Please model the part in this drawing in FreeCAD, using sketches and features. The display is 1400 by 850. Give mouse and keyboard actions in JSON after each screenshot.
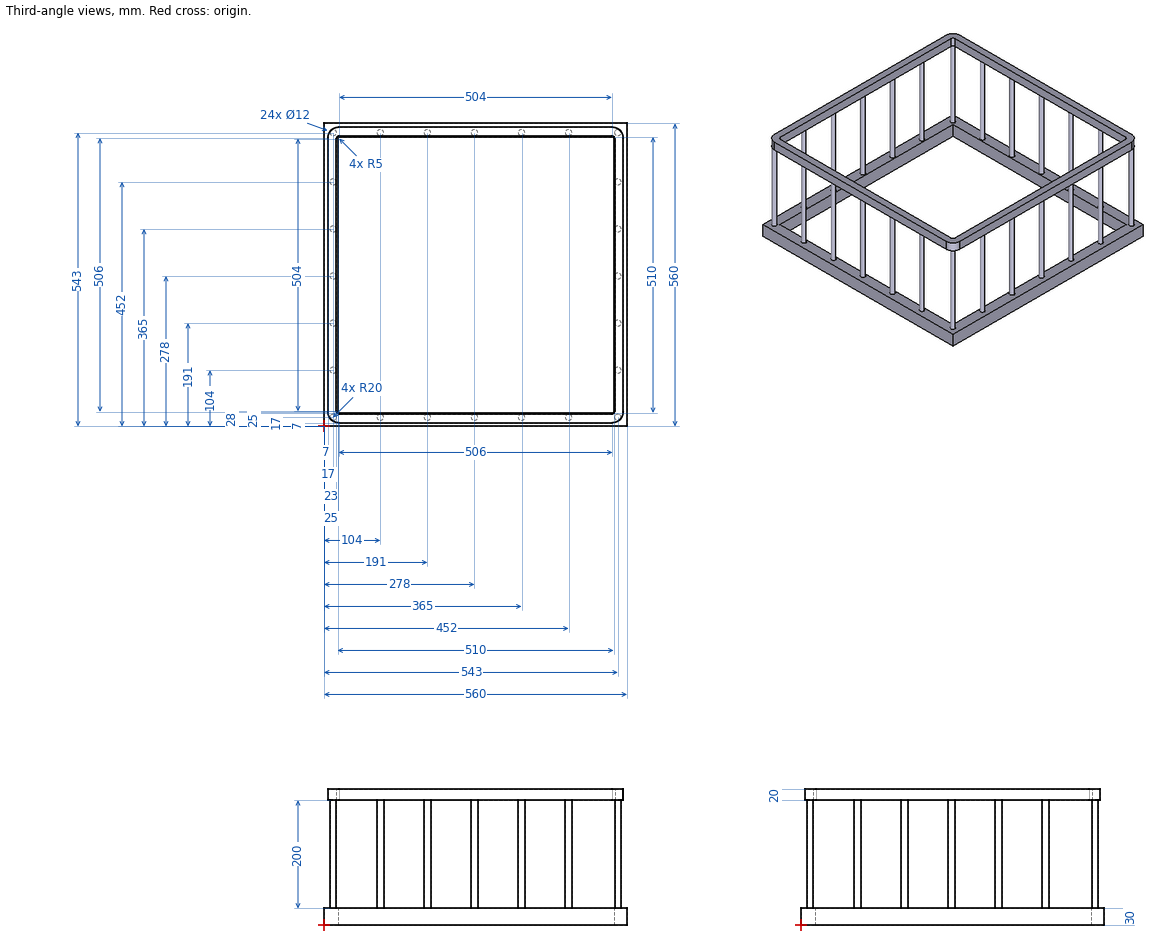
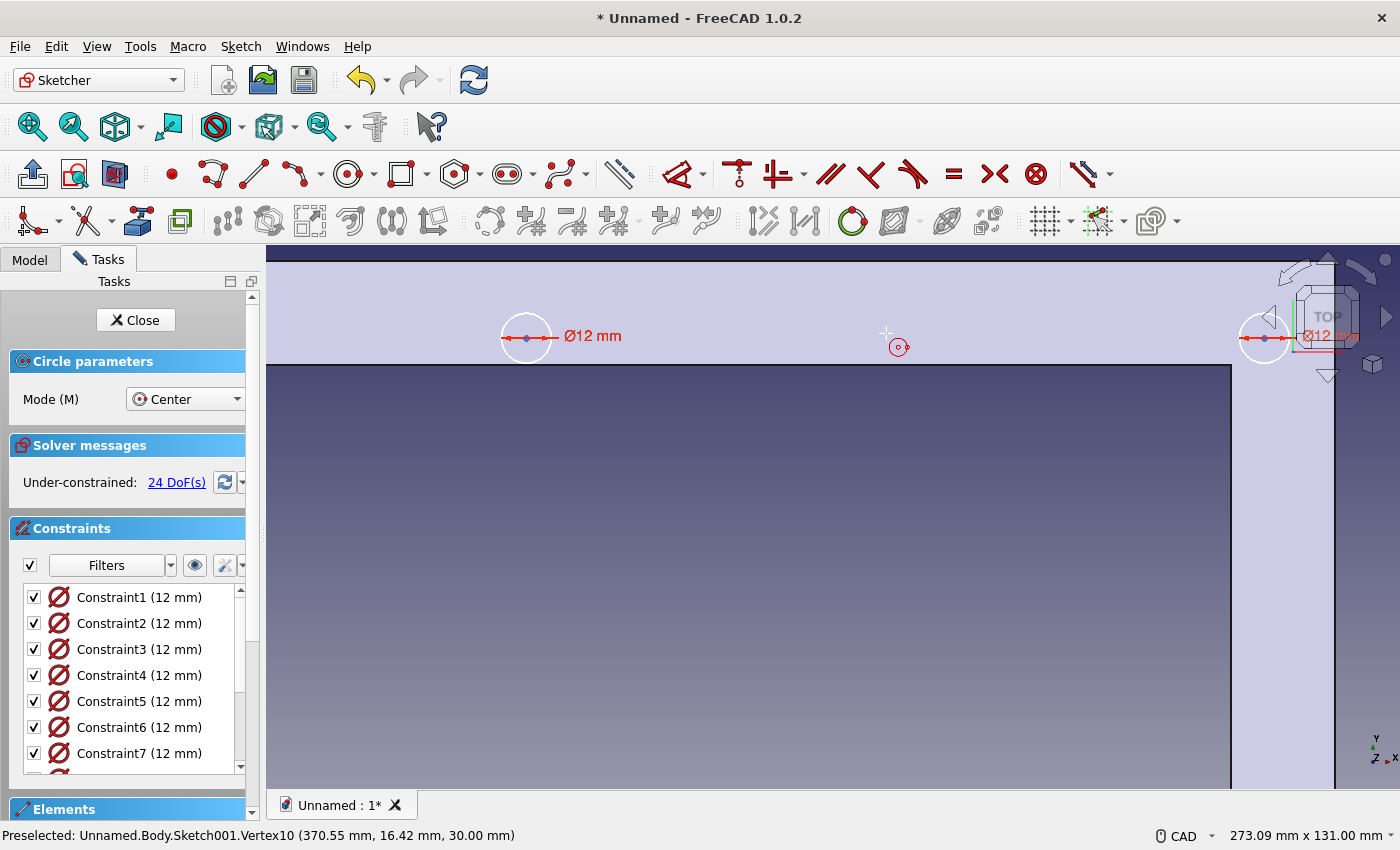
{"action": "scroll", "coordinate": [886, 333], "scroll_direction": "down", "scroll_amount": 9}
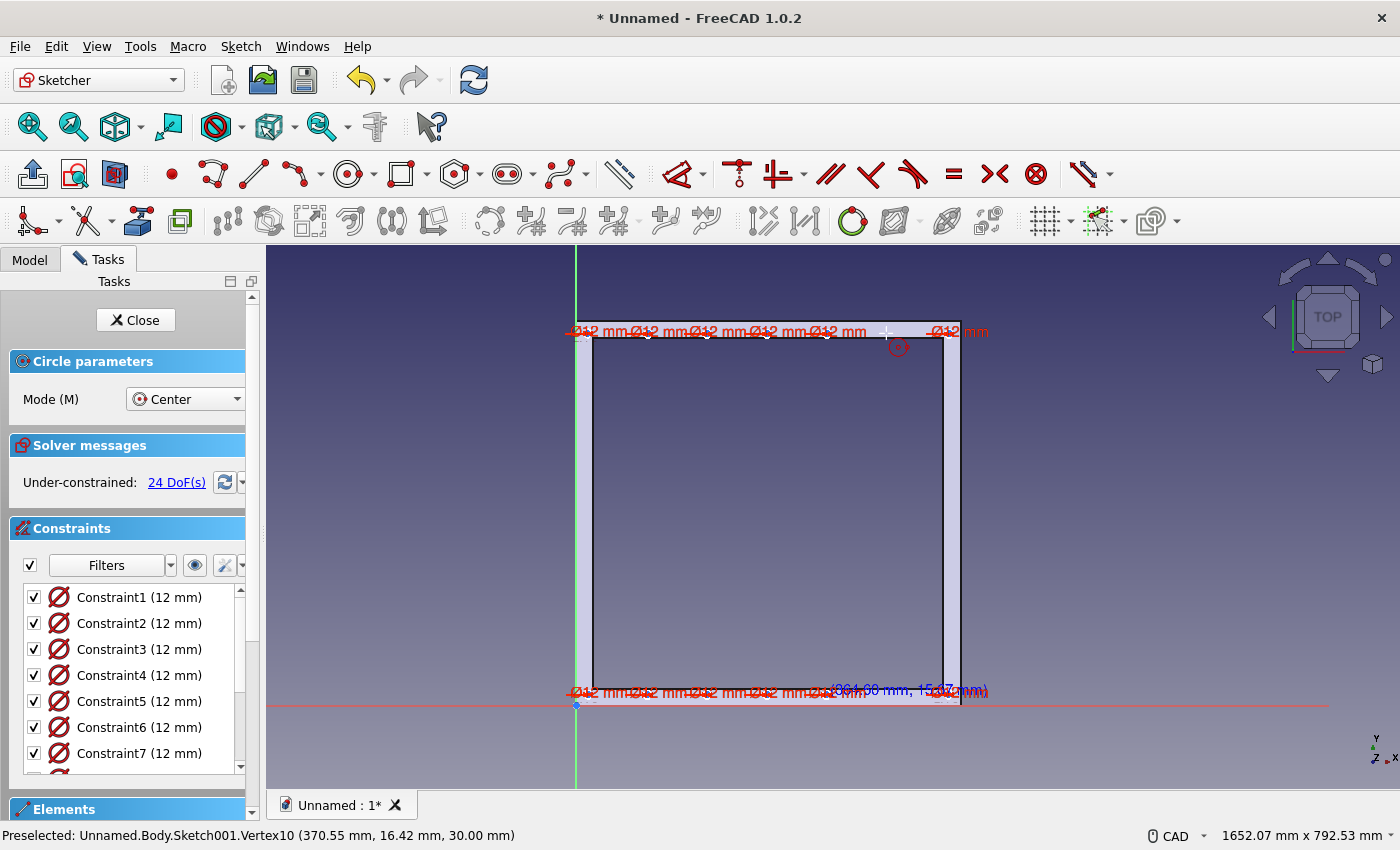
{"action": "left_click", "coordinate": [886, 333]}
{"action": "mouse_move", "coordinate": [889, 330]}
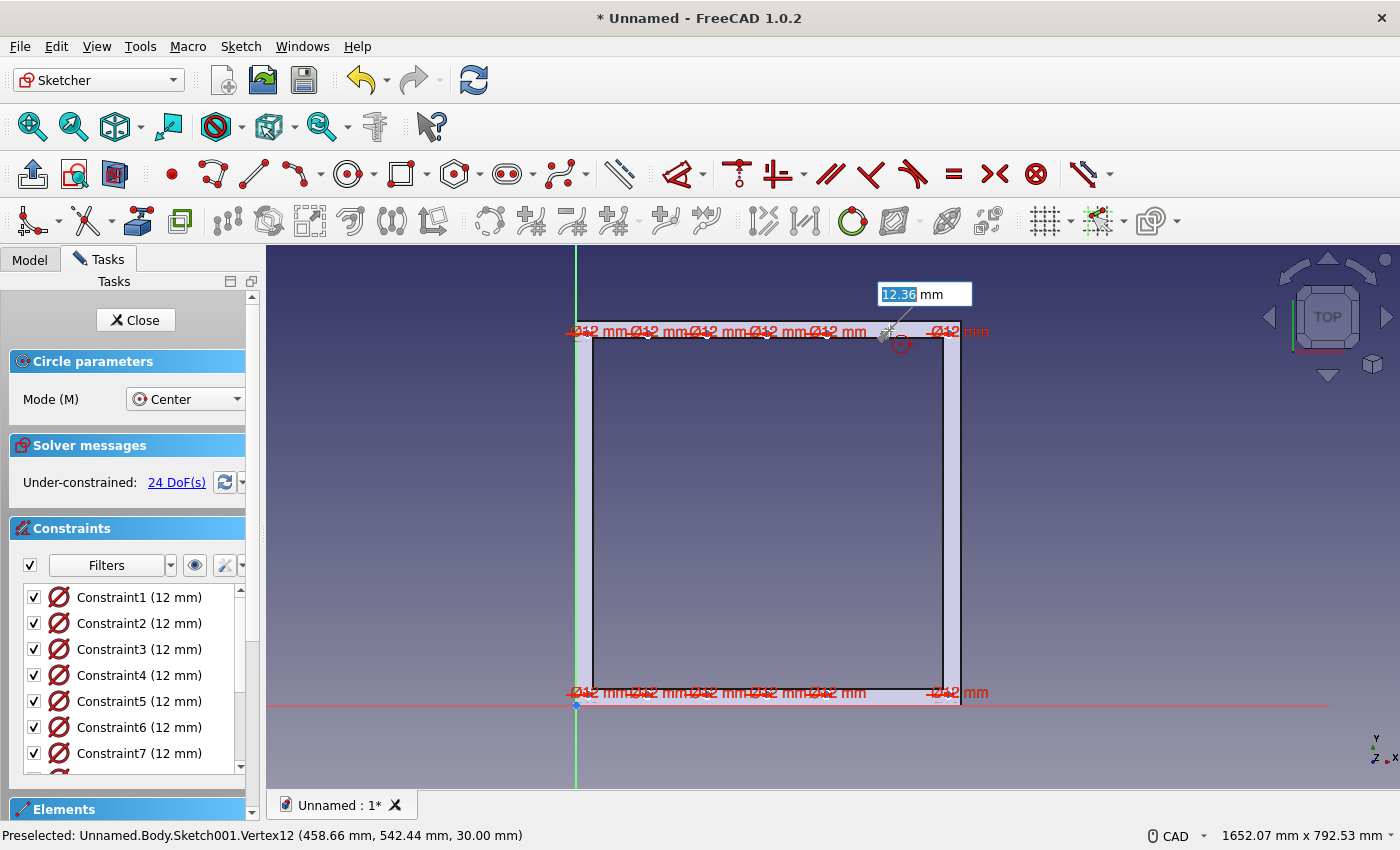
{"action": "type", "text": "12"}
{"action": "key", "text": "Return"}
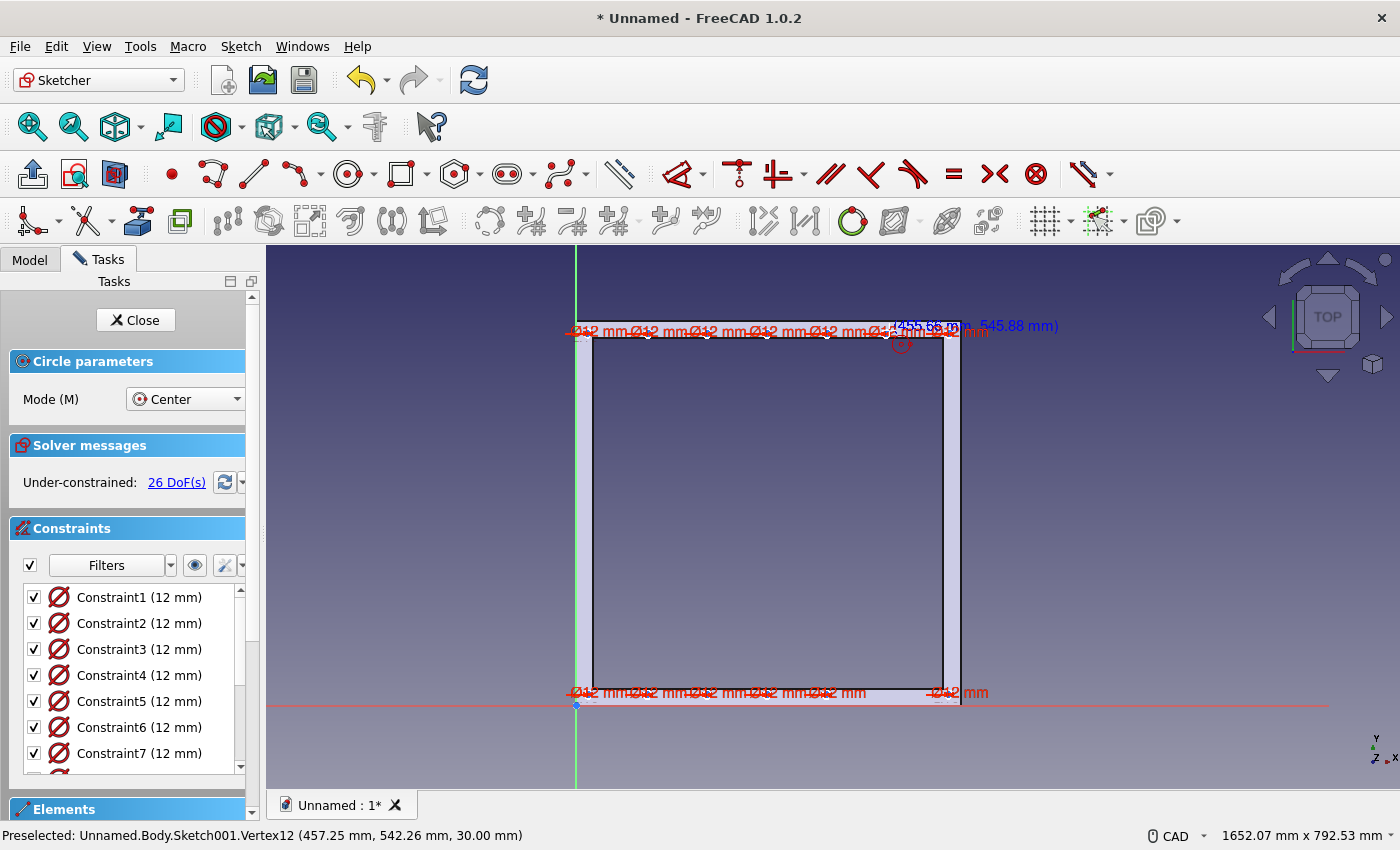
{"action": "scroll", "coordinate": [886, 694], "scroll_direction": "up", "scroll_amount": 9}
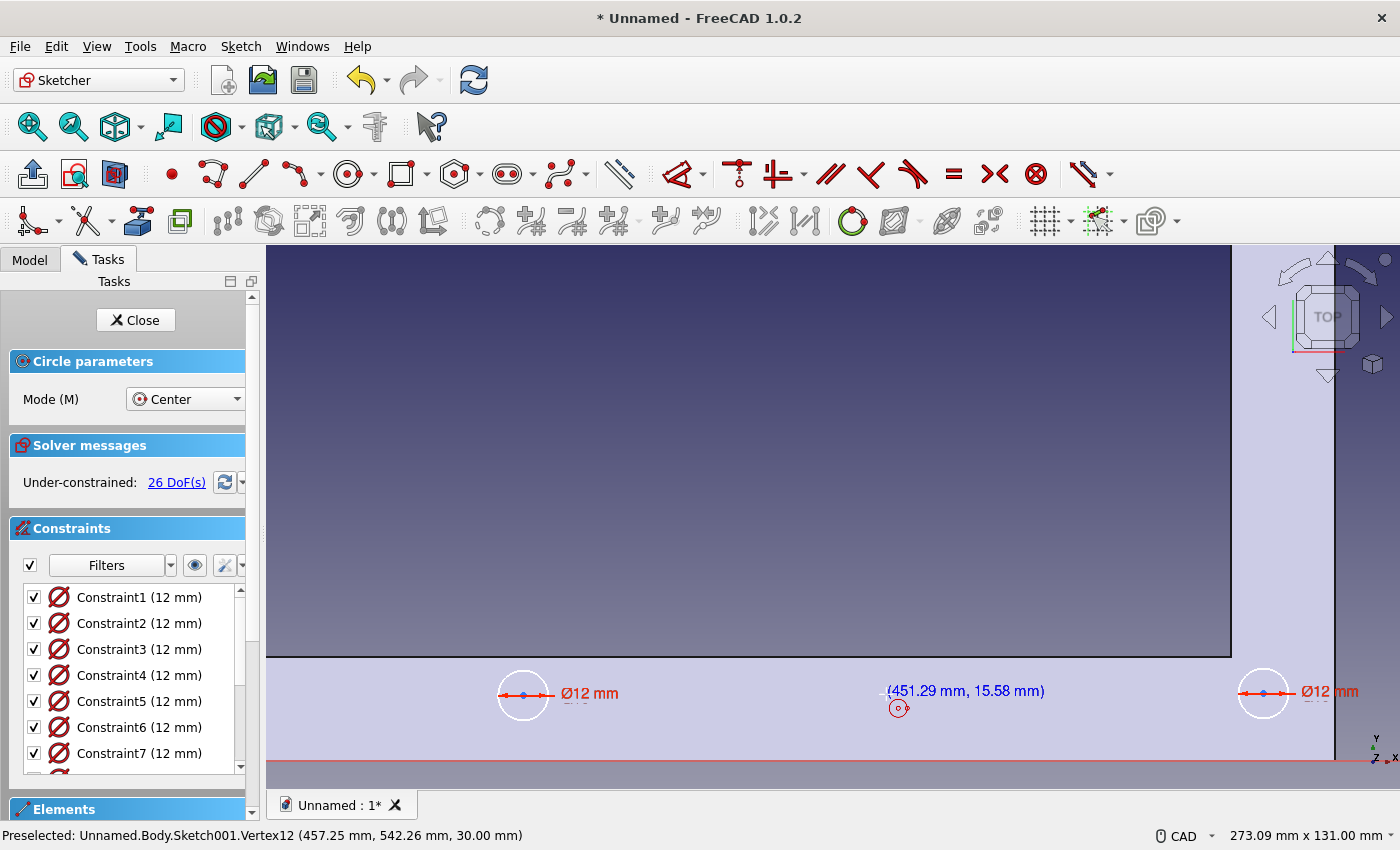
{"action": "scroll", "coordinate": [886, 694], "scroll_direction": "down", "scroll_amount": 9}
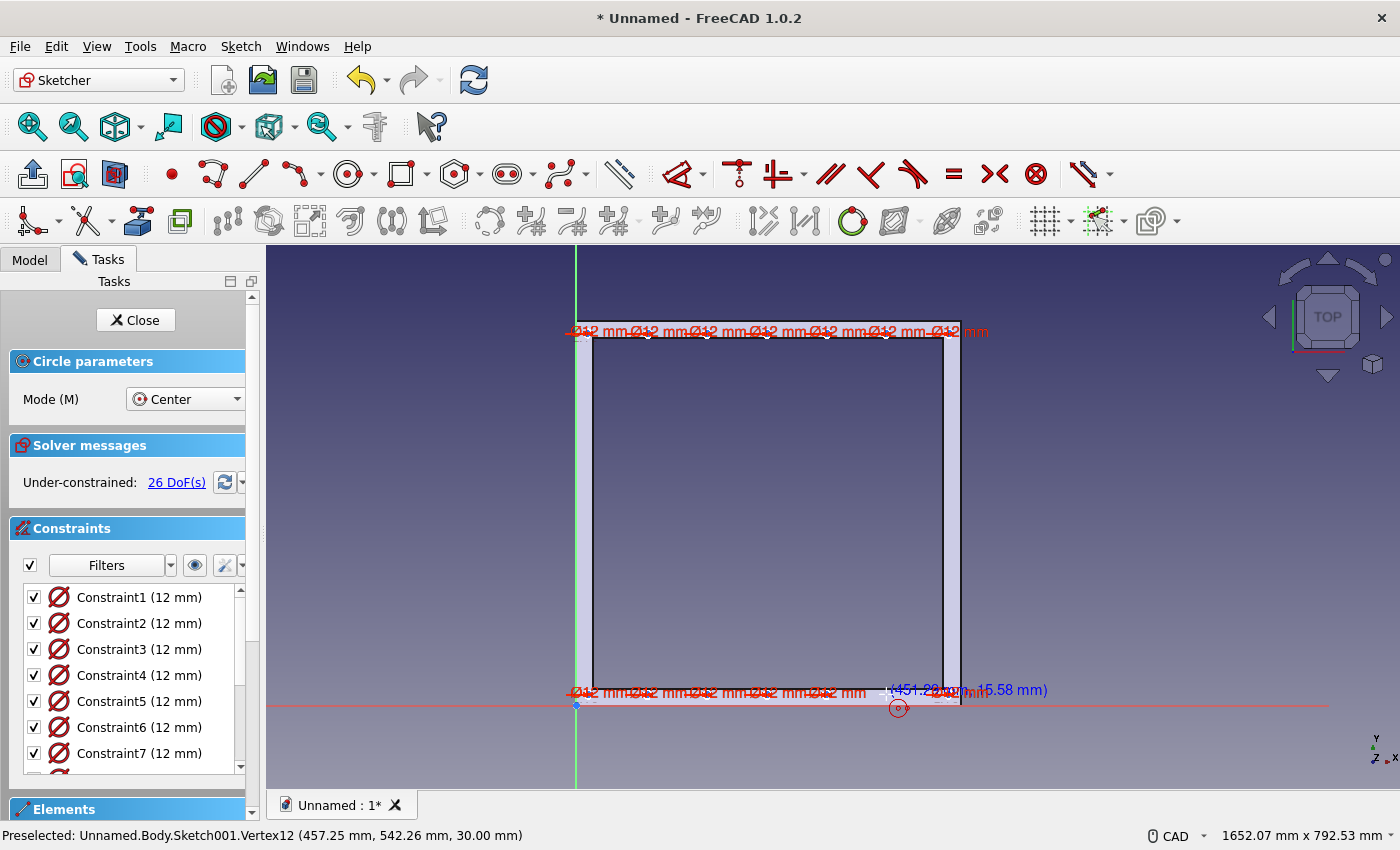
{"action": "scroll", "coordinate": [886, 694], "scroll_direction": "up", "scroll_amount": 2}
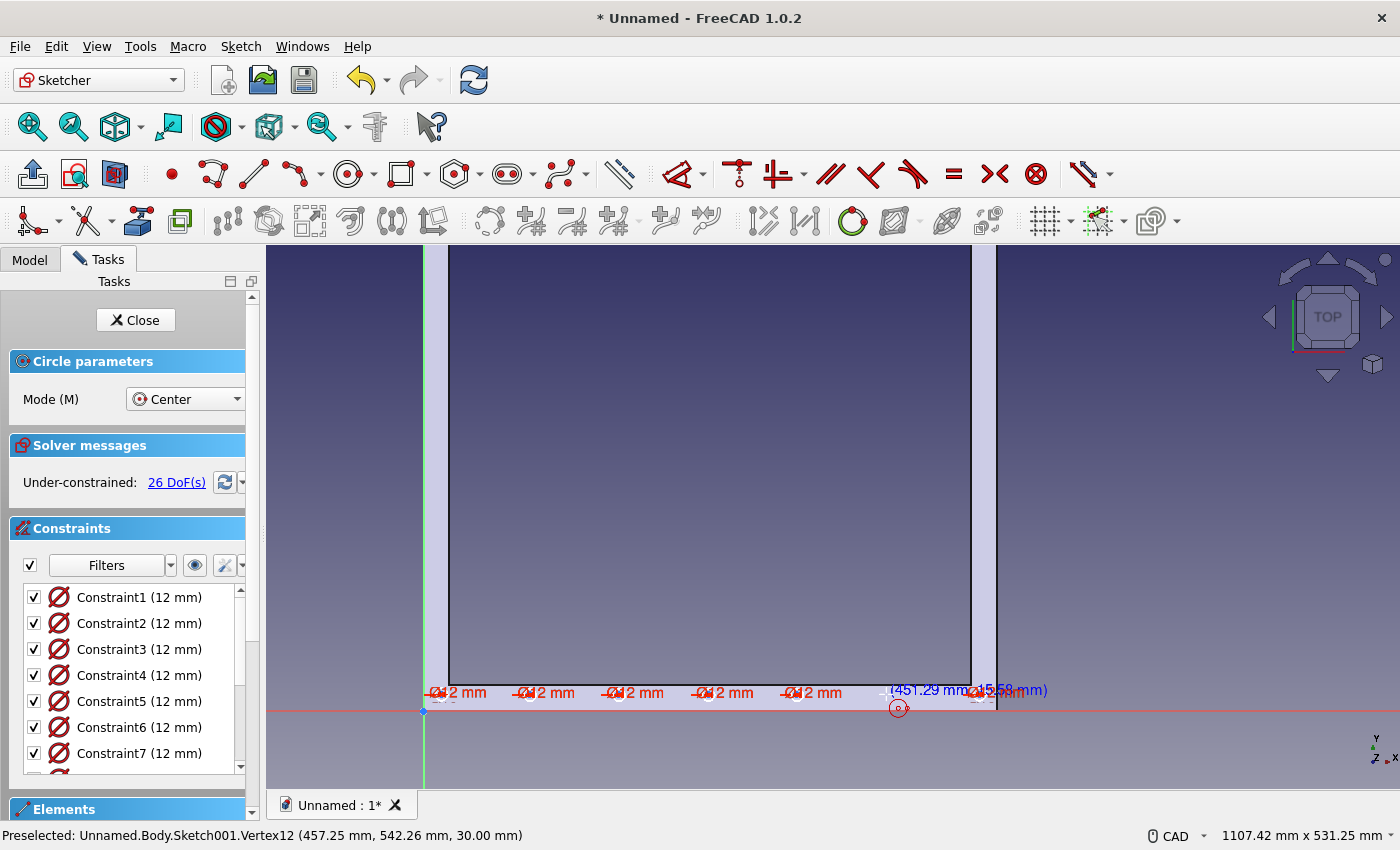
{"action": "left_click", "coordinate": [886, 694]}
{"action": "mouse_move", "coordinate": [891, 689]}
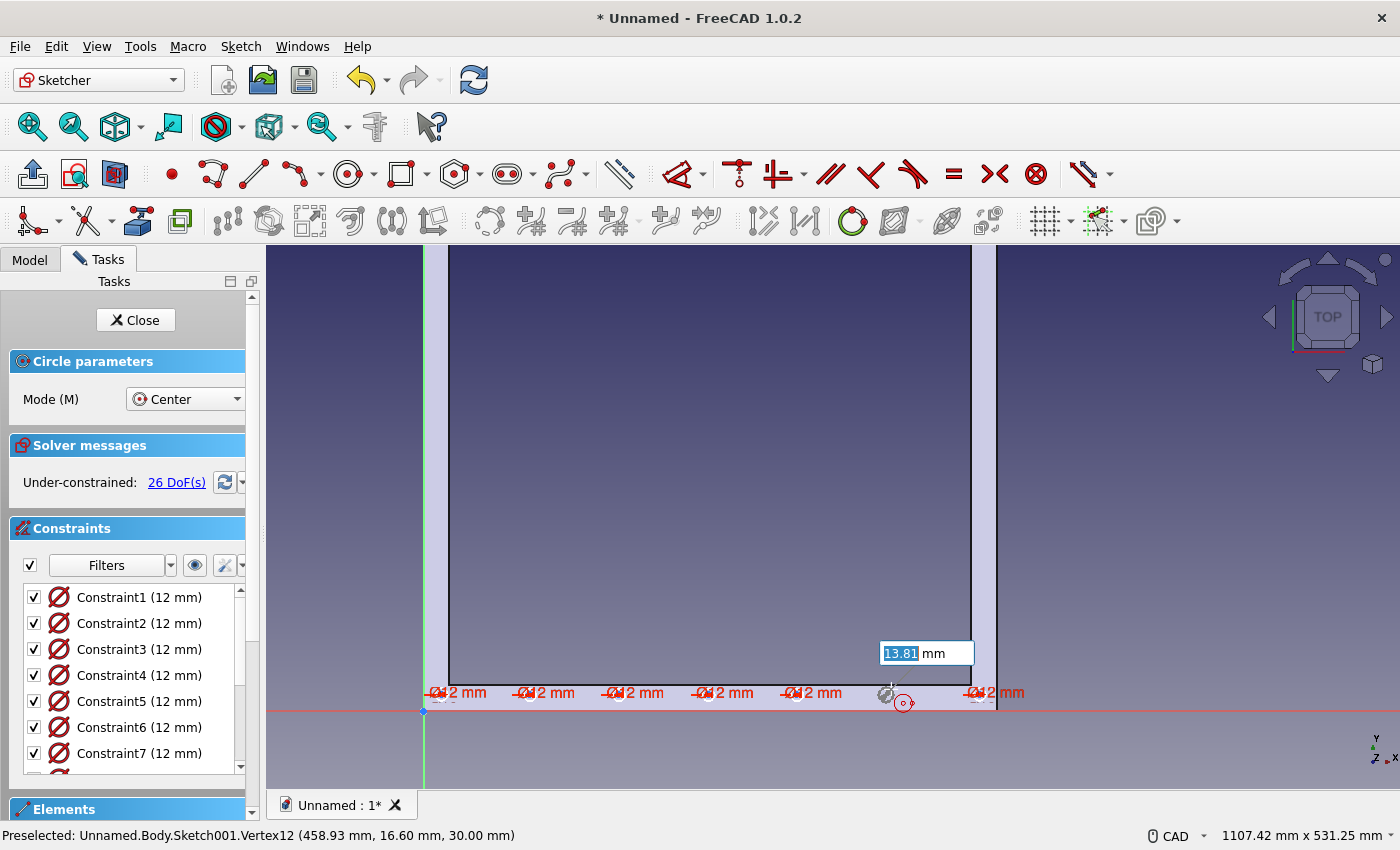
{"action": "type", "text": "12"}
{"action": "key", "text": "Return"}